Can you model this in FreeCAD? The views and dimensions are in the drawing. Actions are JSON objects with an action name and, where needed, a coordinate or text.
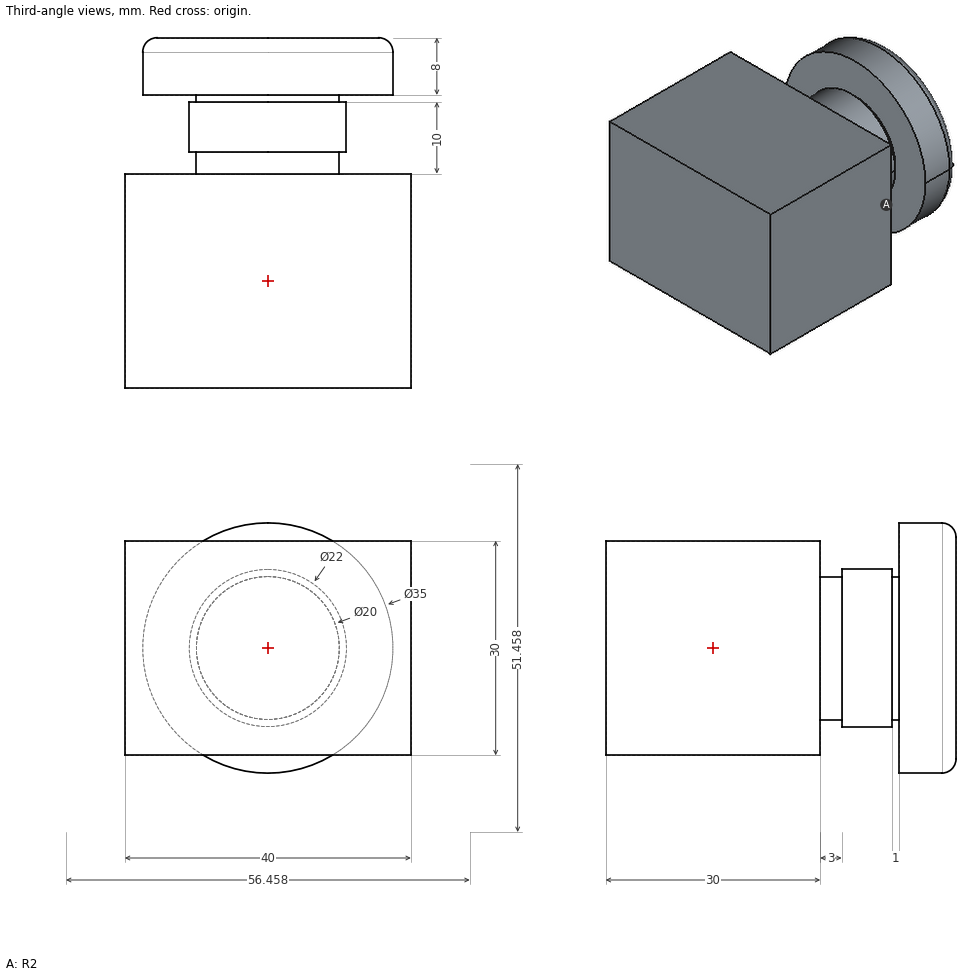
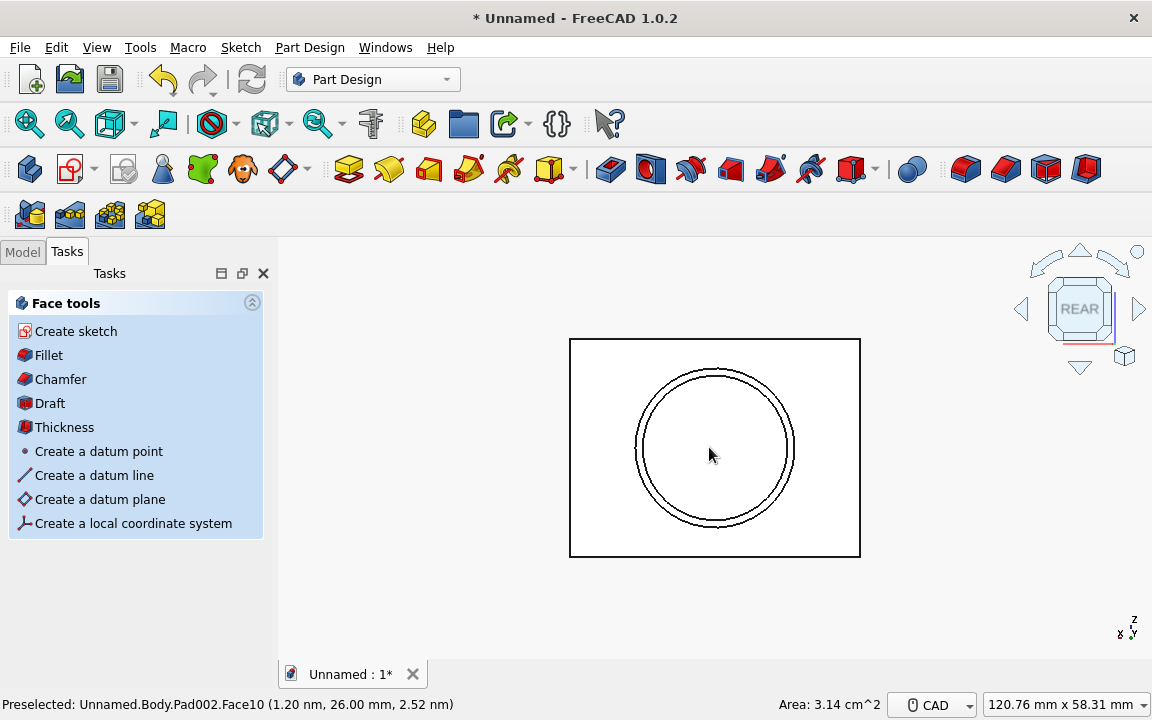
{"action": "left_click", "coordinate": [70, 170]}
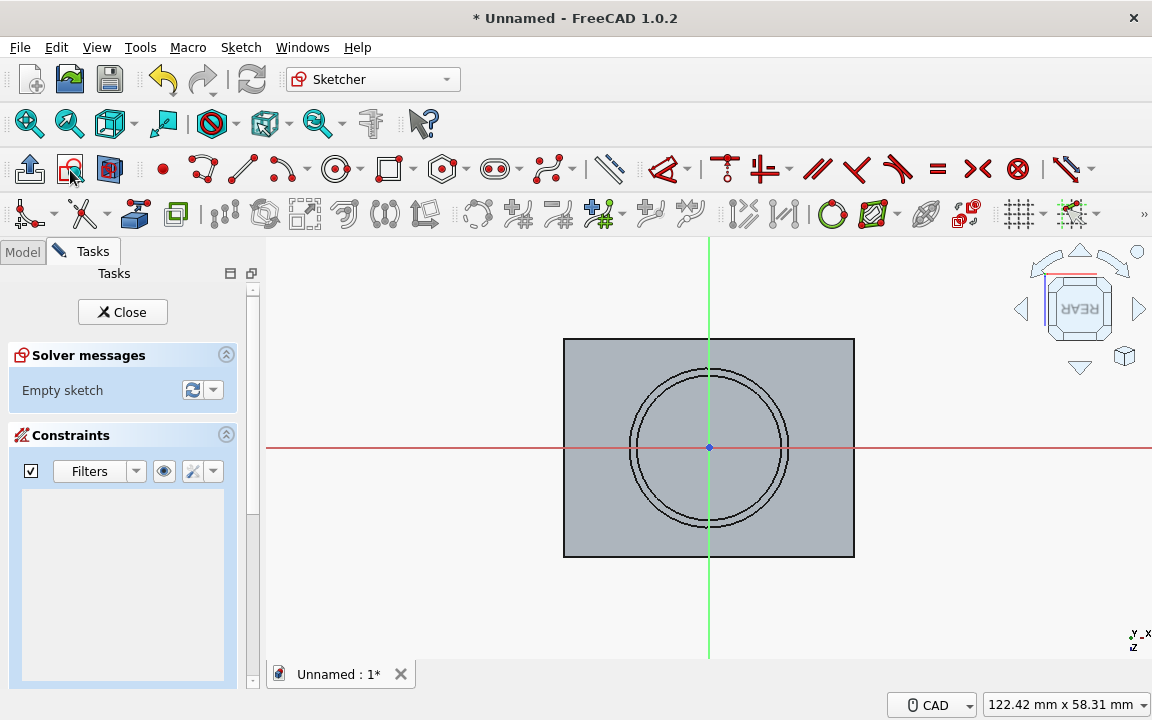
{"action": "left_click", "coordinate": [336, 170]}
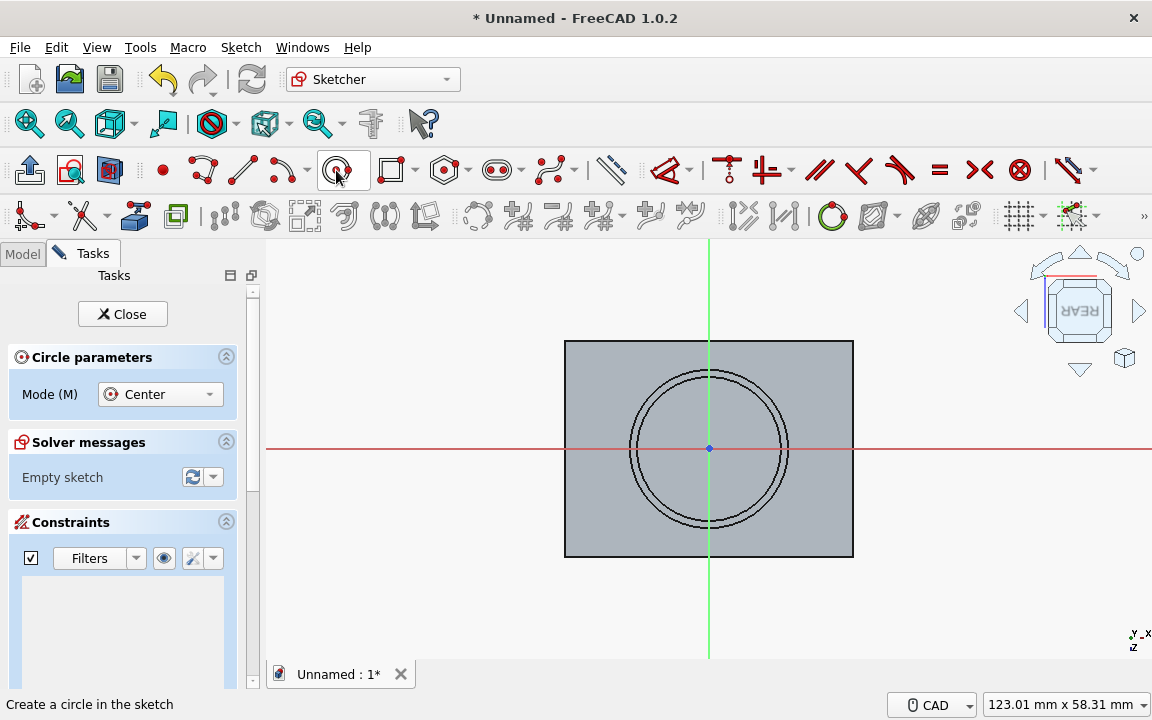
{"action": "left_click", "coordinate": [709, 449]}
{"action": "mouse_move", "coordinate": [798, 360]}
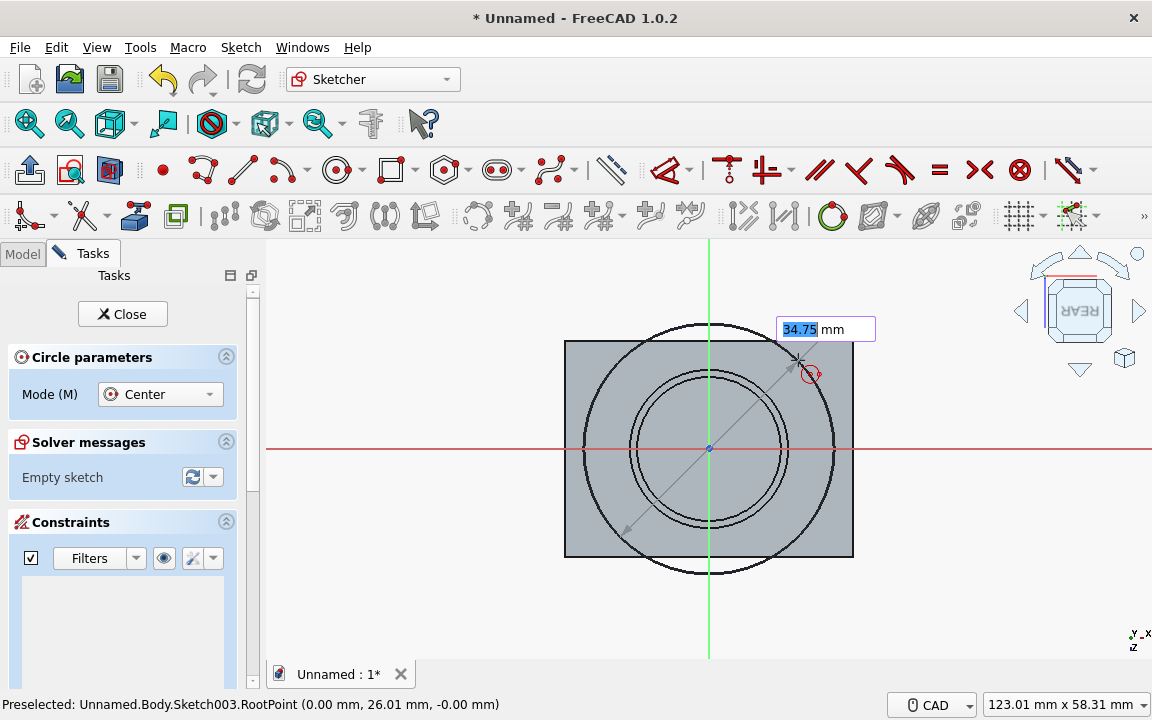
{"action": "type", "text": "35"}
{"action": "key", "text": "Return"}
{"action": "key", "text": "Escape"}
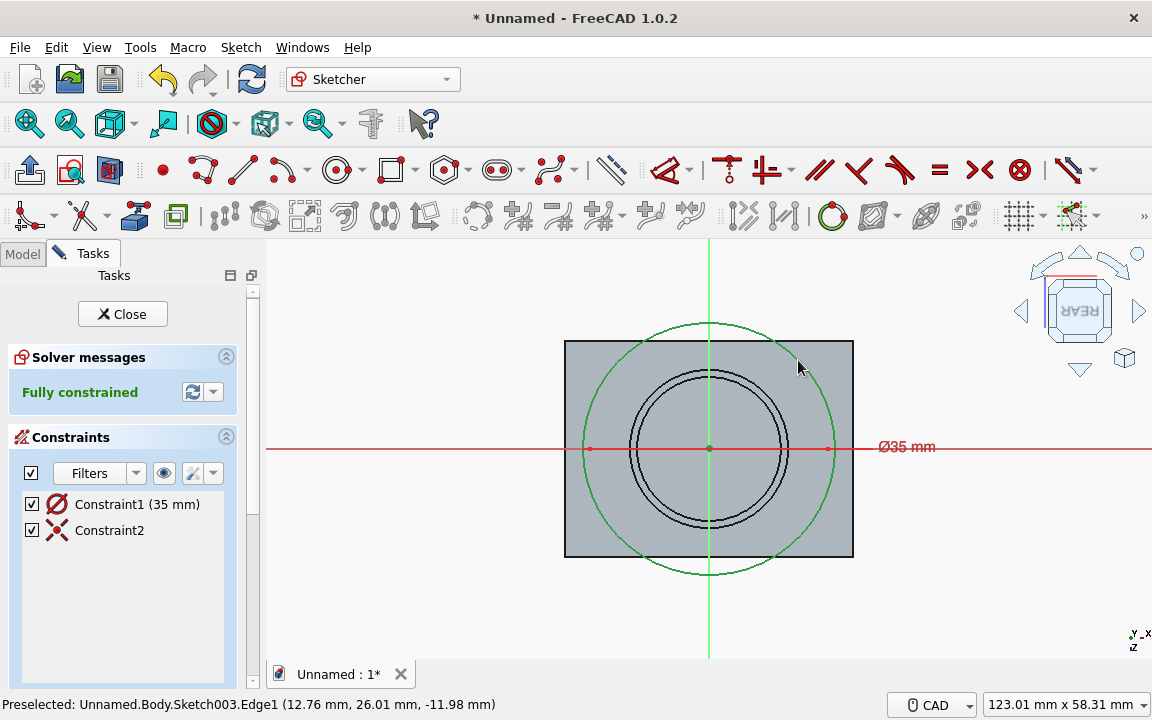
{"action": "left_click", "coordinate": [123, 314]}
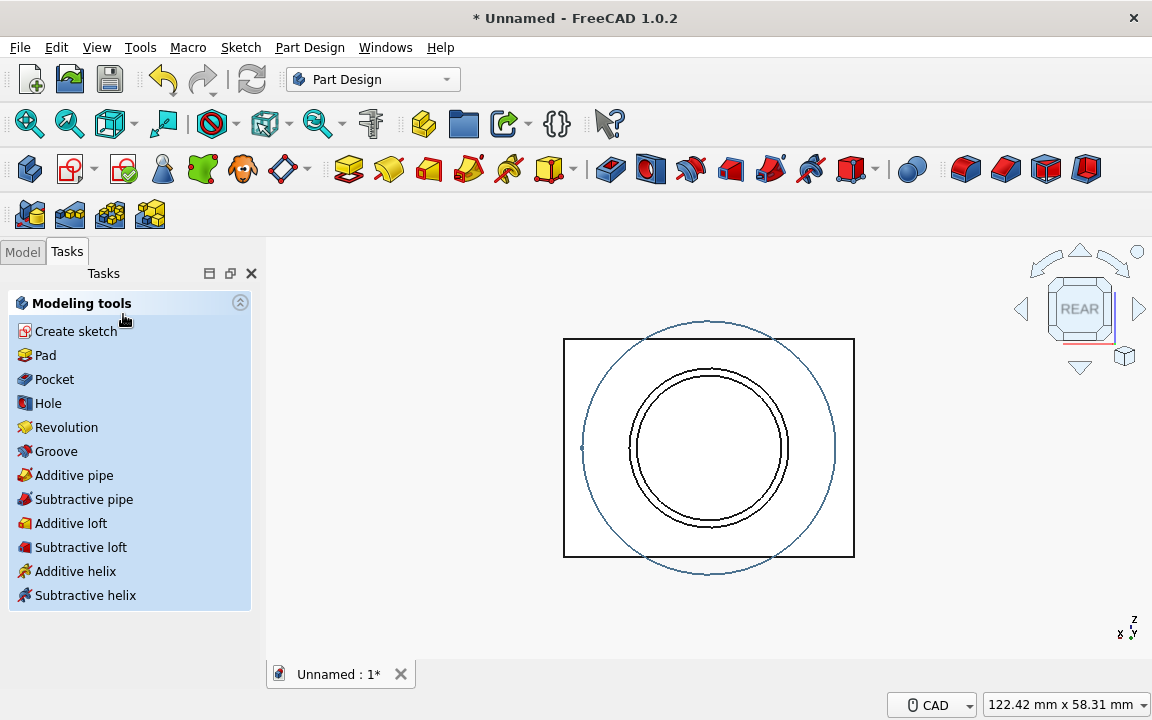
{"action": "left_click", "coordinate": [350, 170]}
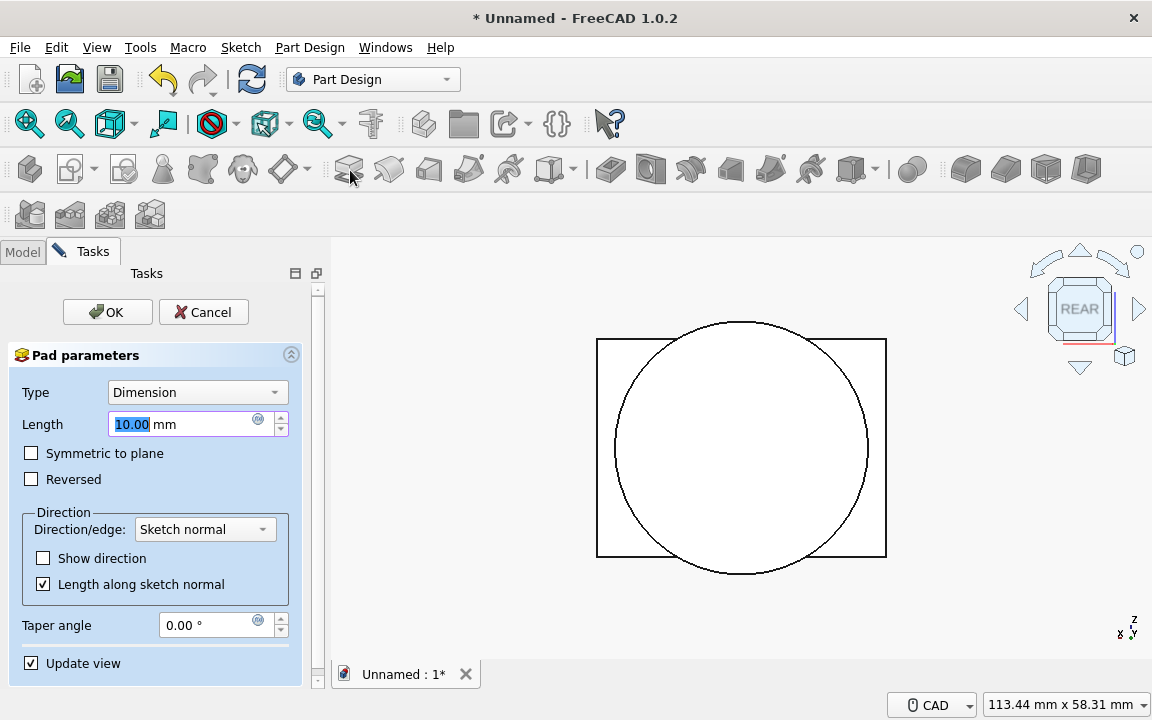
{"action": "type", "text": "8"}
{"action": "key", "text": "Tab"}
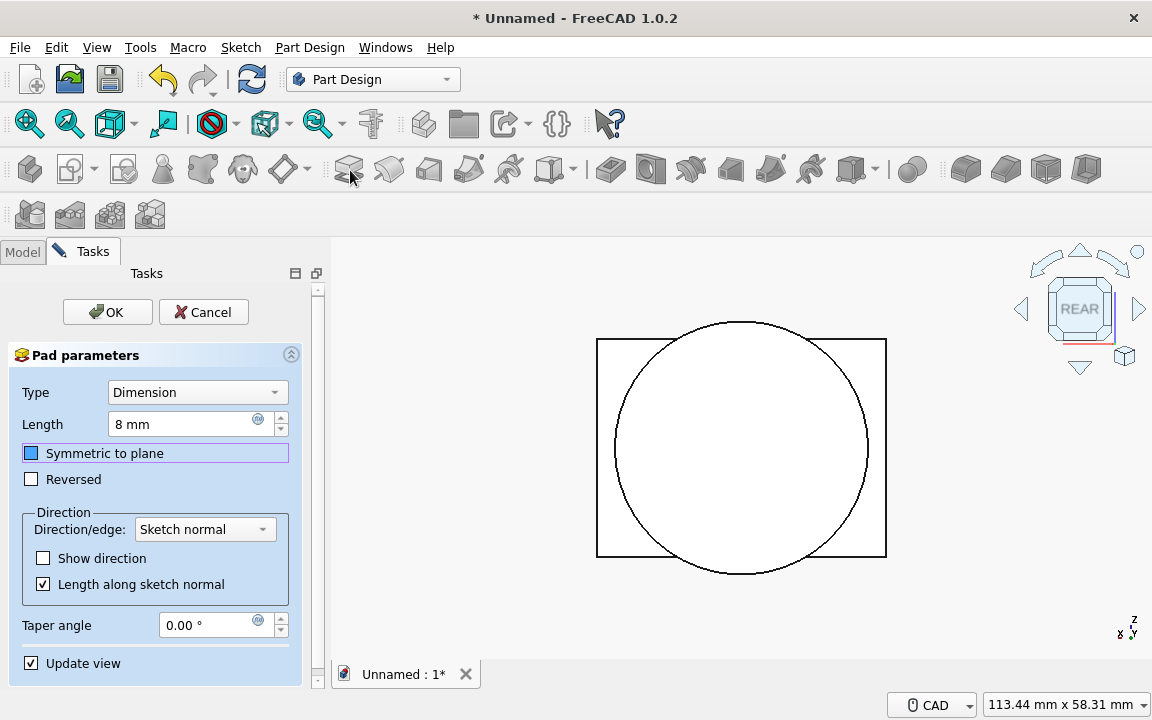
{"action": "left_click", "coordinate": [108, 312]}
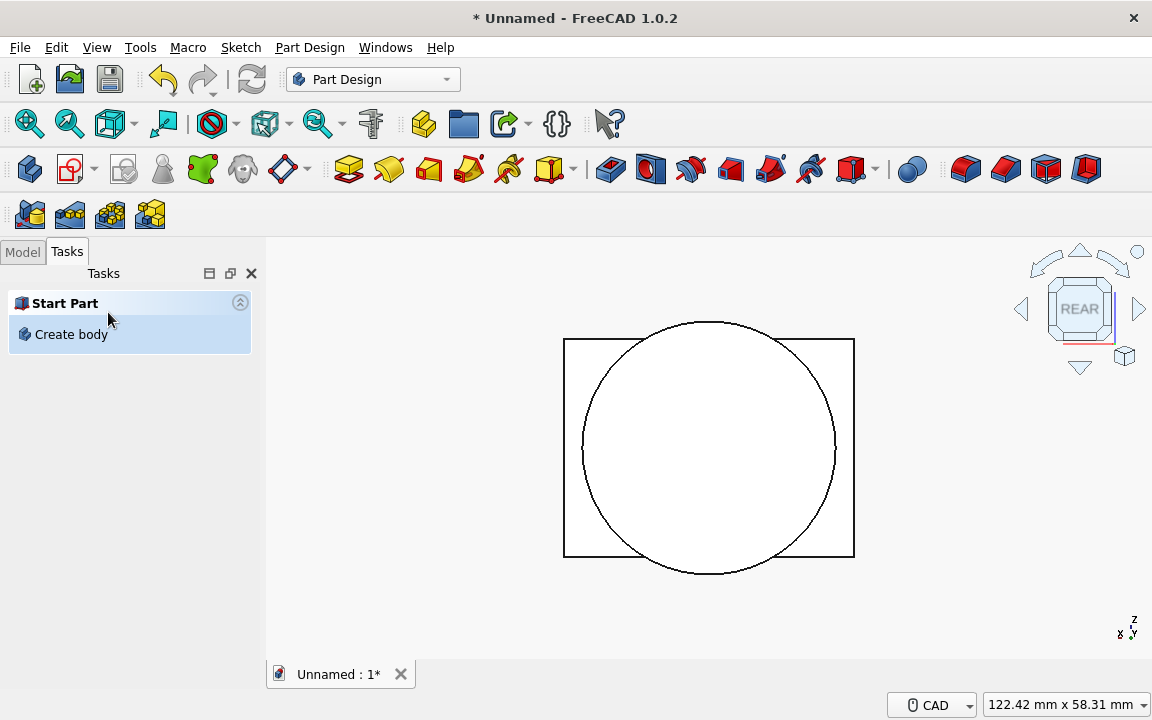
{"action": "left_click", "coordinate": [836, 447]}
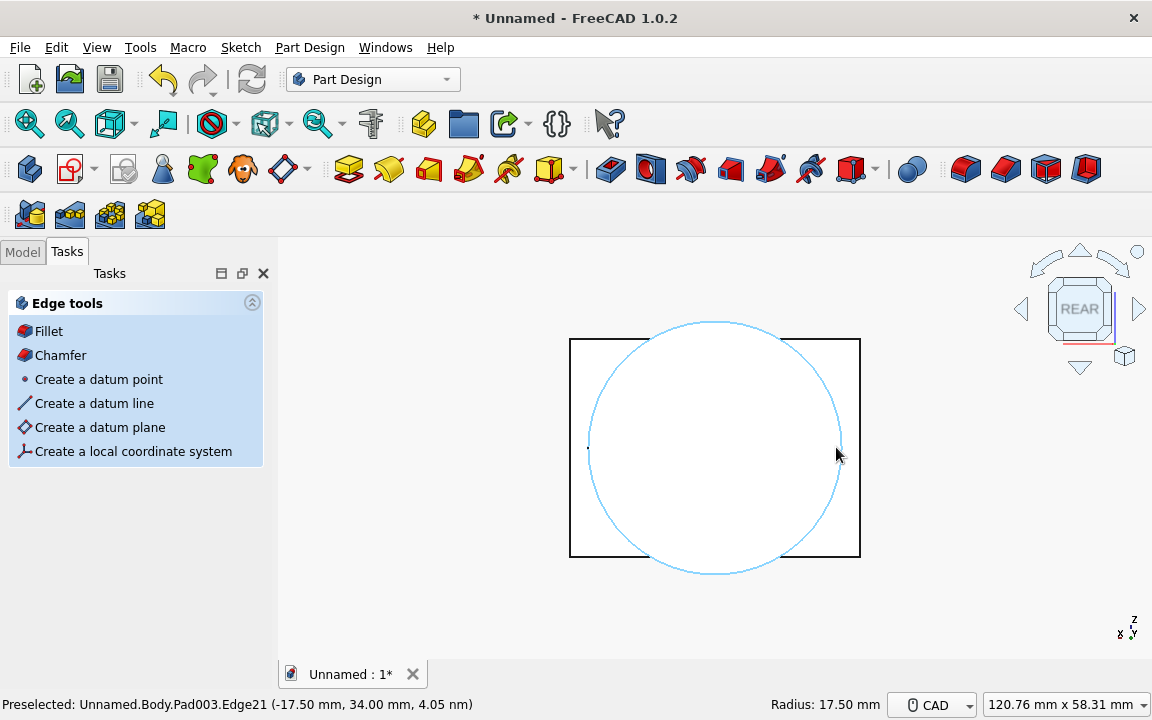
{"action": "left_click", "coordinate": [966, 170]}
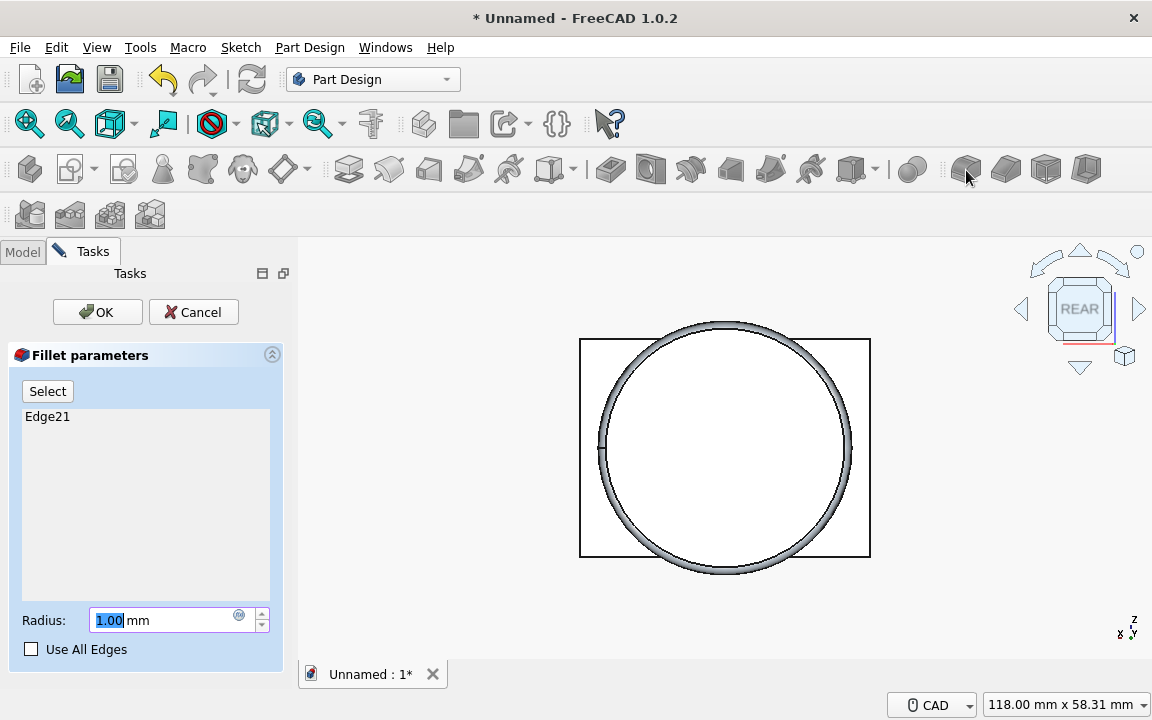
{"action": "type", "text": "2"}
{"action": "key", "text": "Tab"}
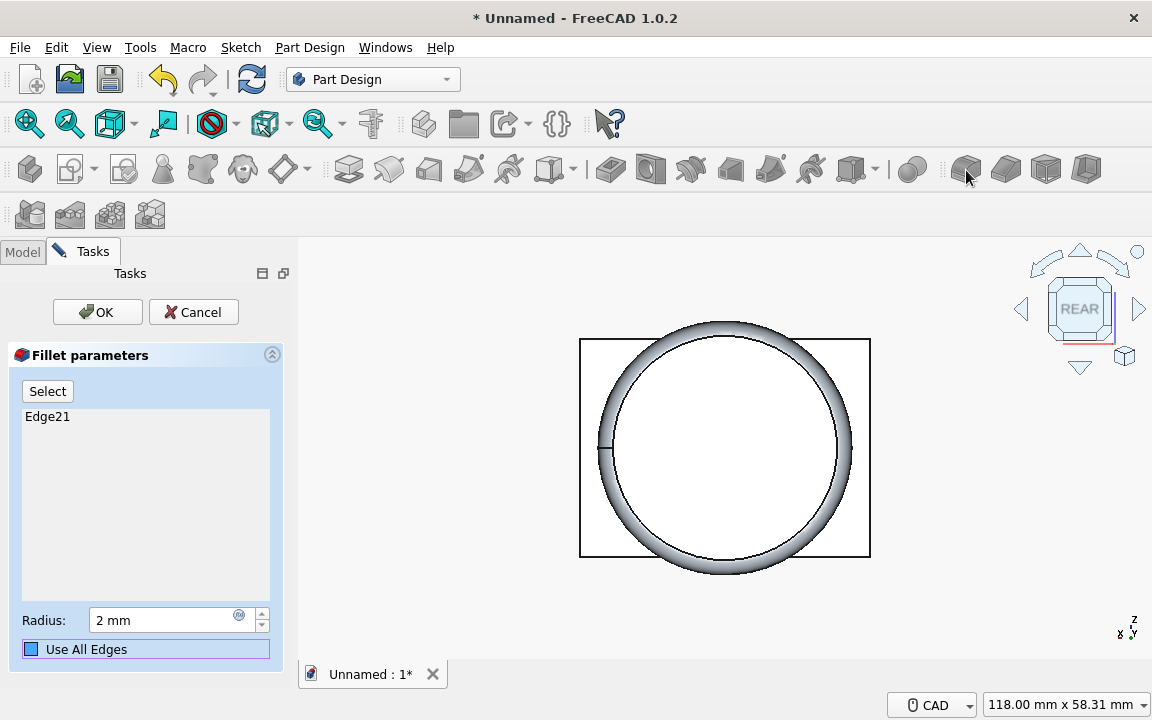
{"action": "left_click", "coordinate": [98, 312]}